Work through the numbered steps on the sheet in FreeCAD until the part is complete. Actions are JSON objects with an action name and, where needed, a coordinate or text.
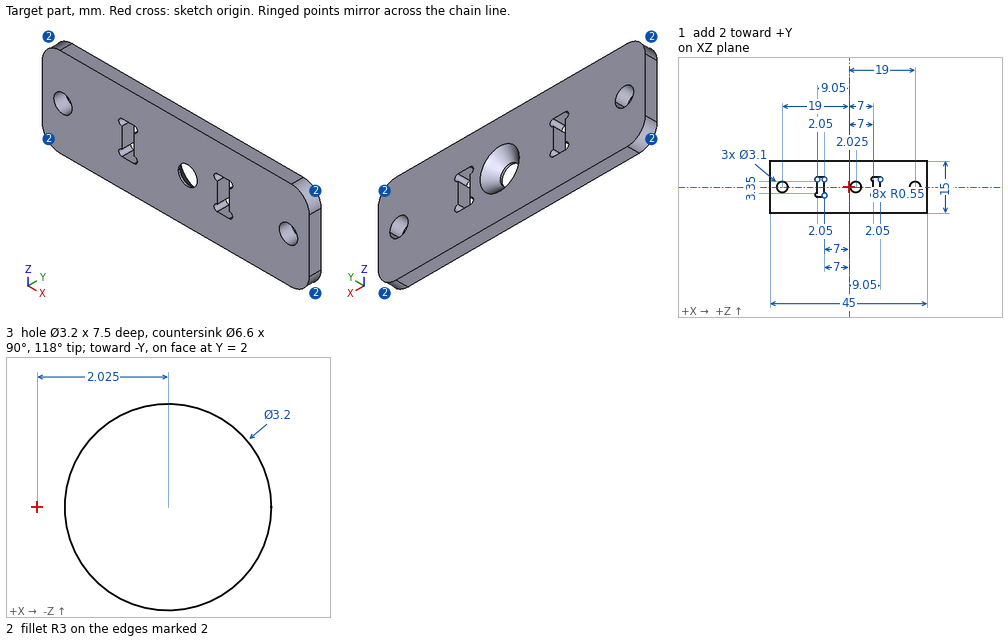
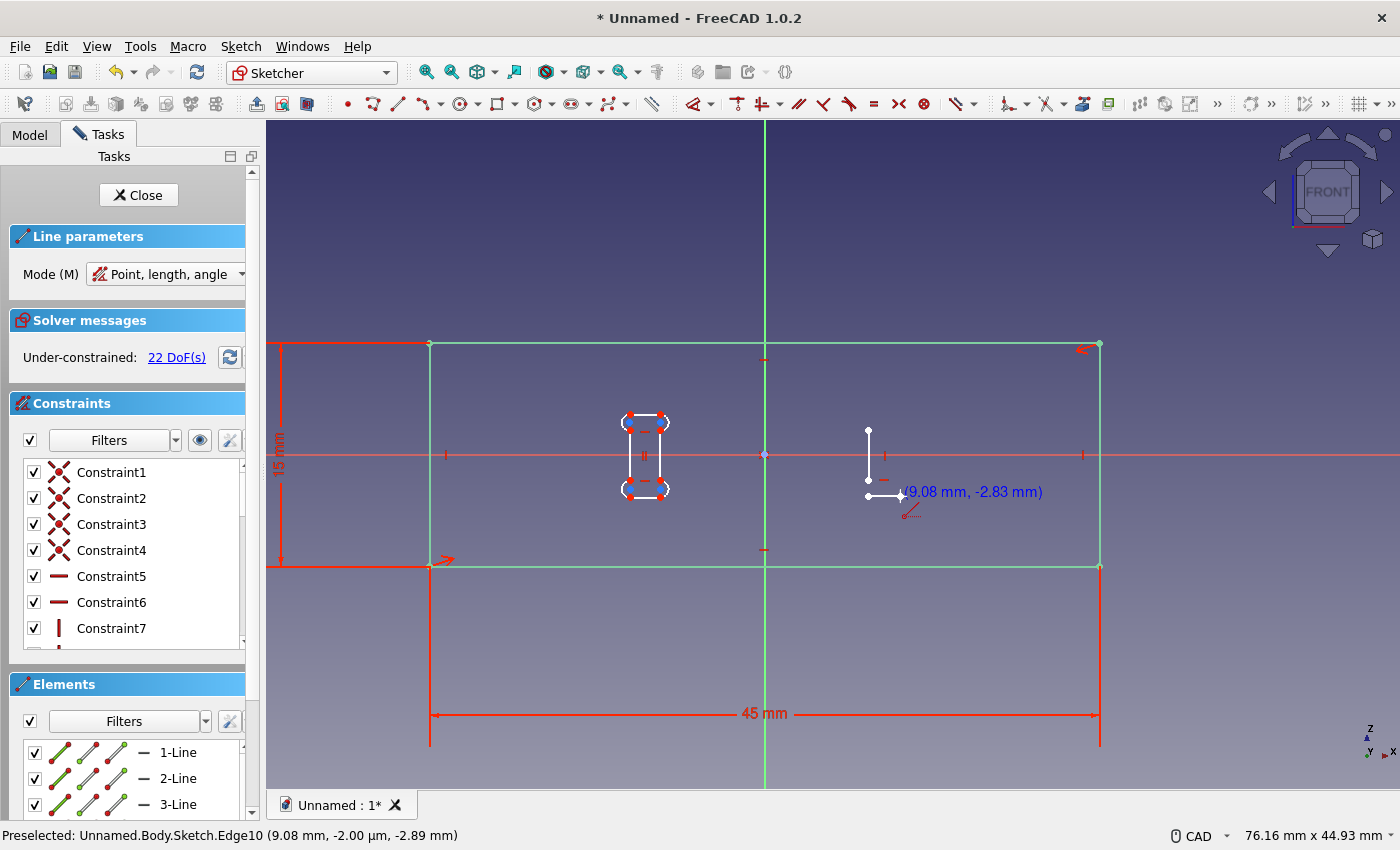
{"action": "left_click", "coordinate": [900, 480]}
{"action": "left_click", "coordinate": [900, 430]}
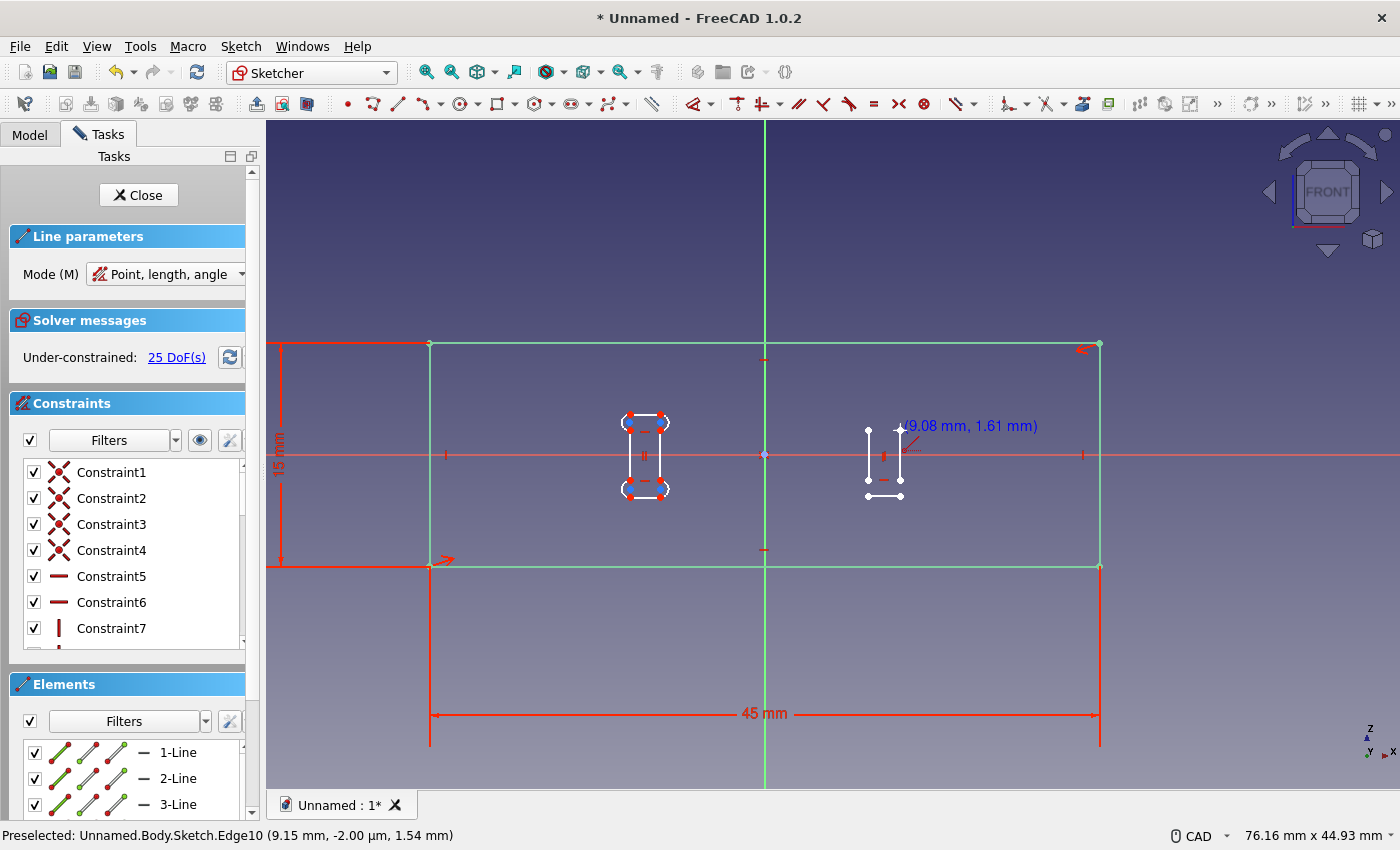
{"action": "left_click", "coordinate": [900, 414]}
{"action": "left_click", "coordinate": [869, 414]}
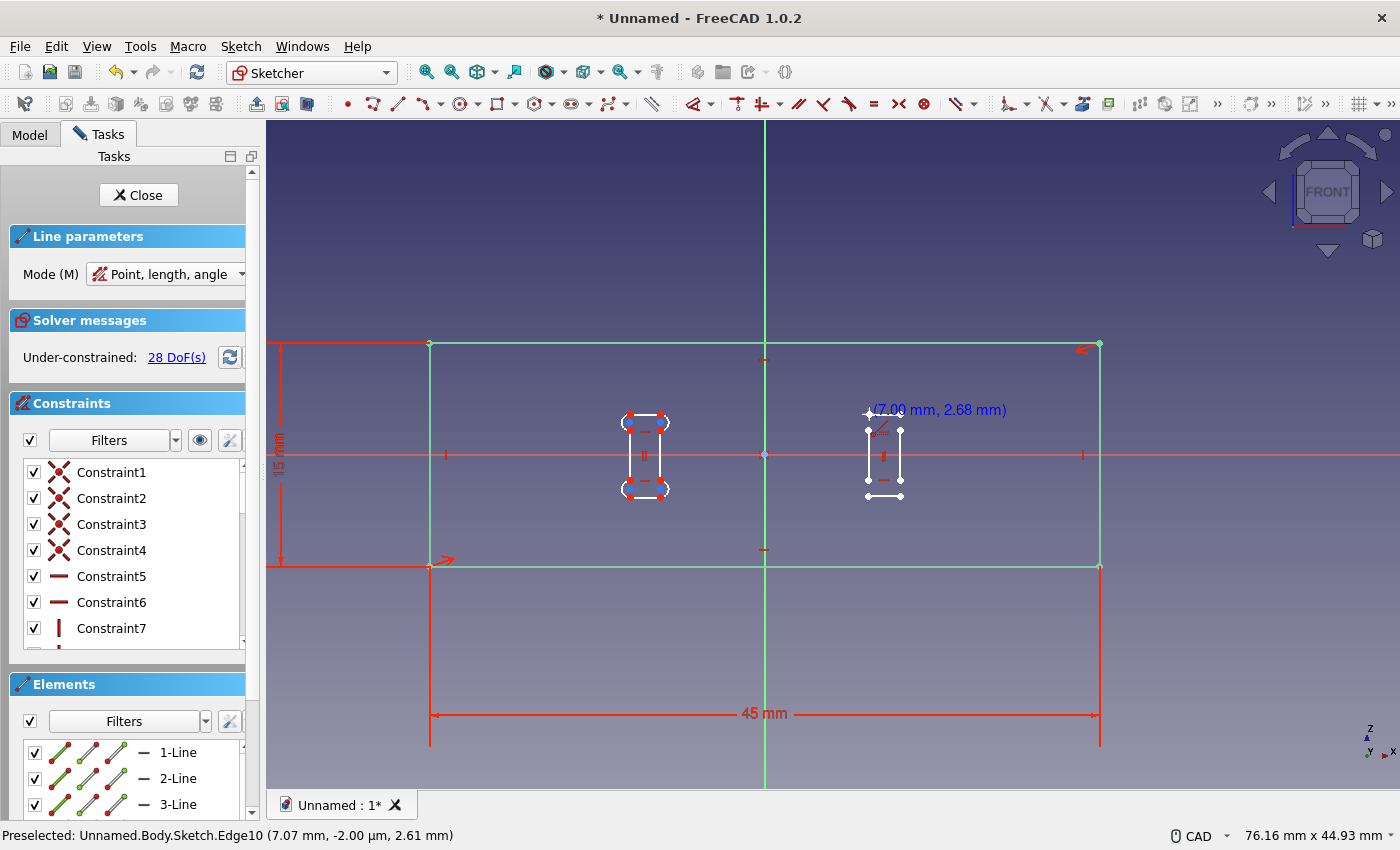
{"action": "left_click", "coordinate": [422, 104]}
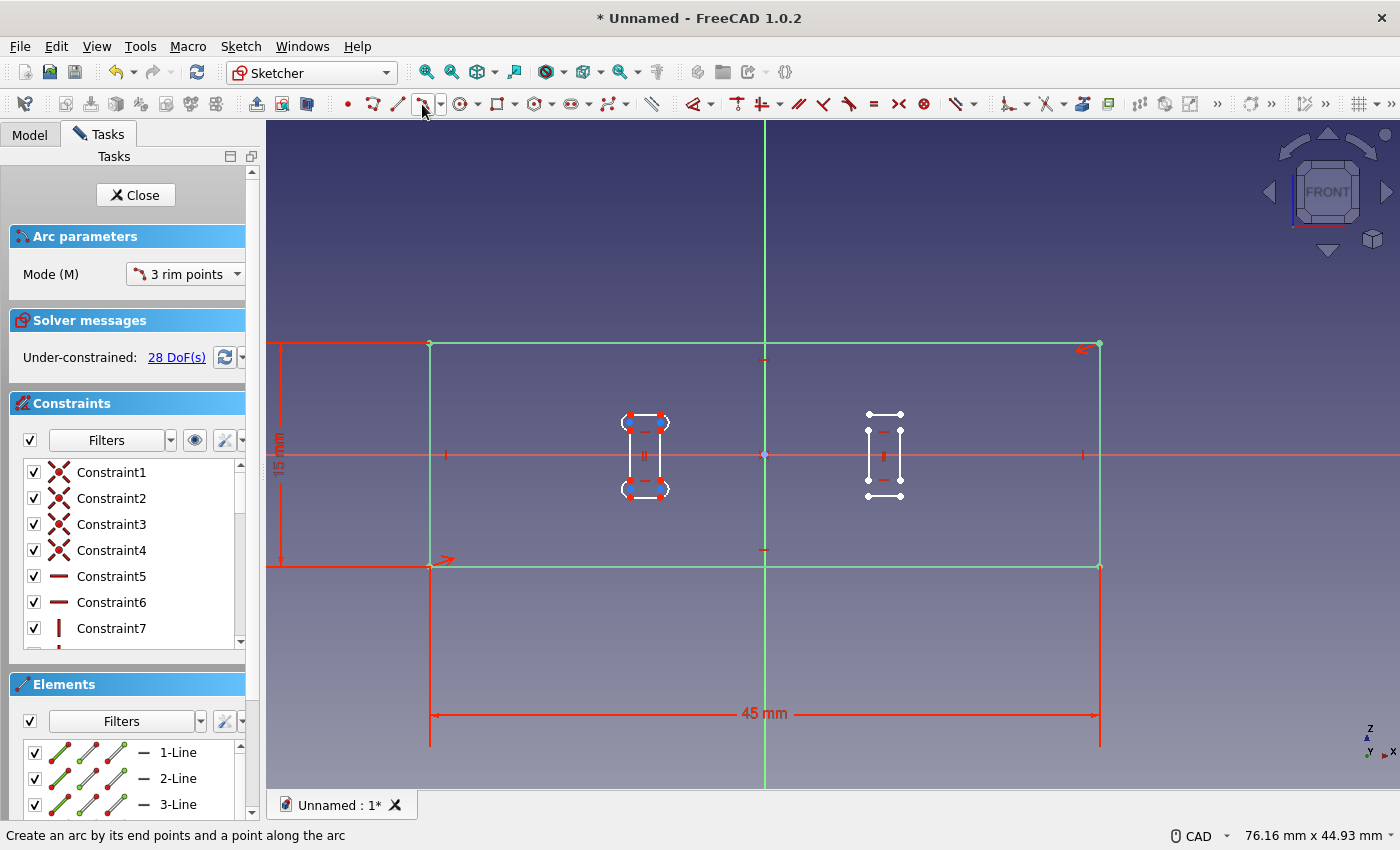
{"action": "left_click", "coordinate": [869, 480]}
{"action": "left_click", "coordinate": [869, 496]}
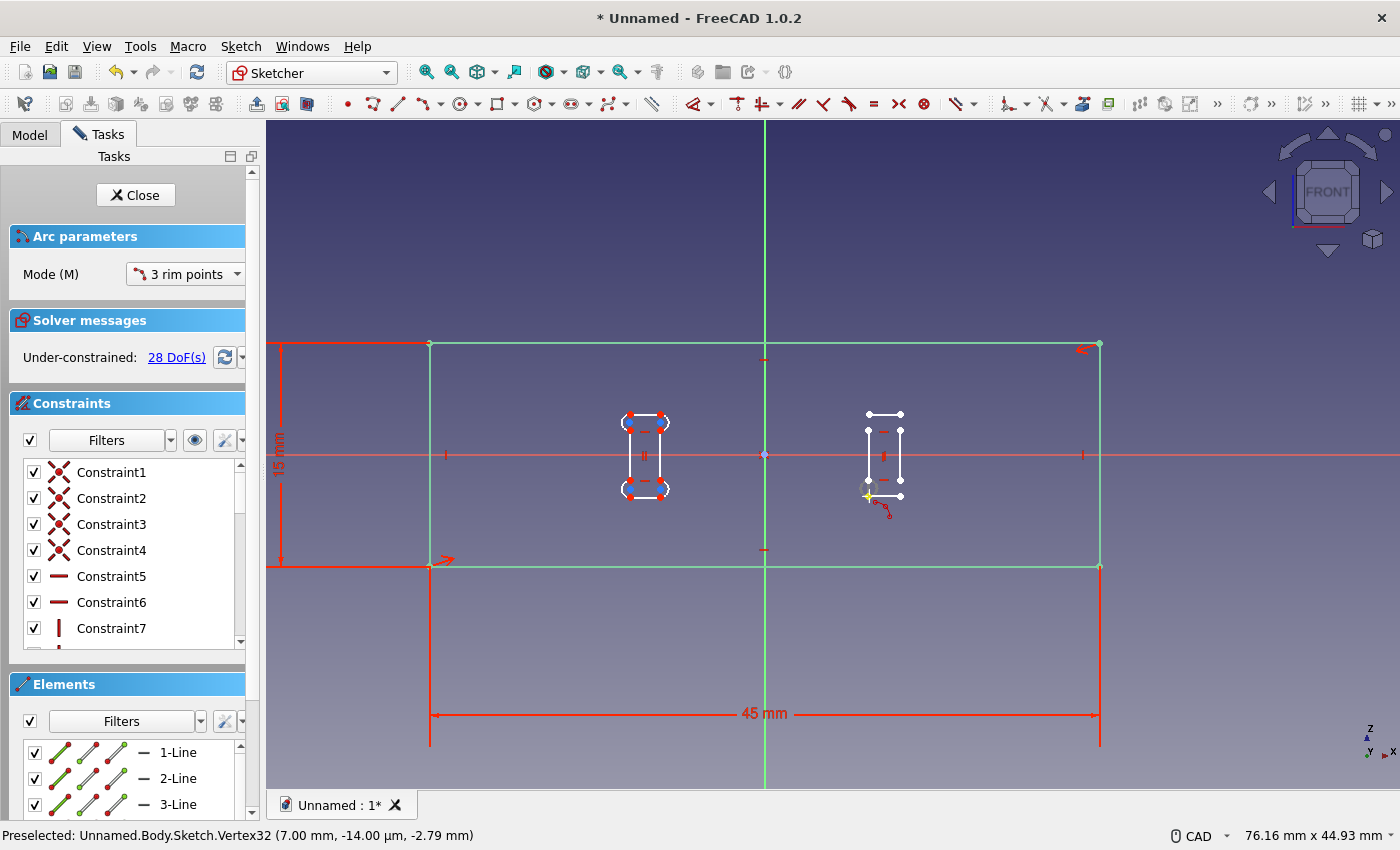
{"action": "scroll", "coordinate": [861, 488], "scroll_direction": "up", "scroll_amount": 4}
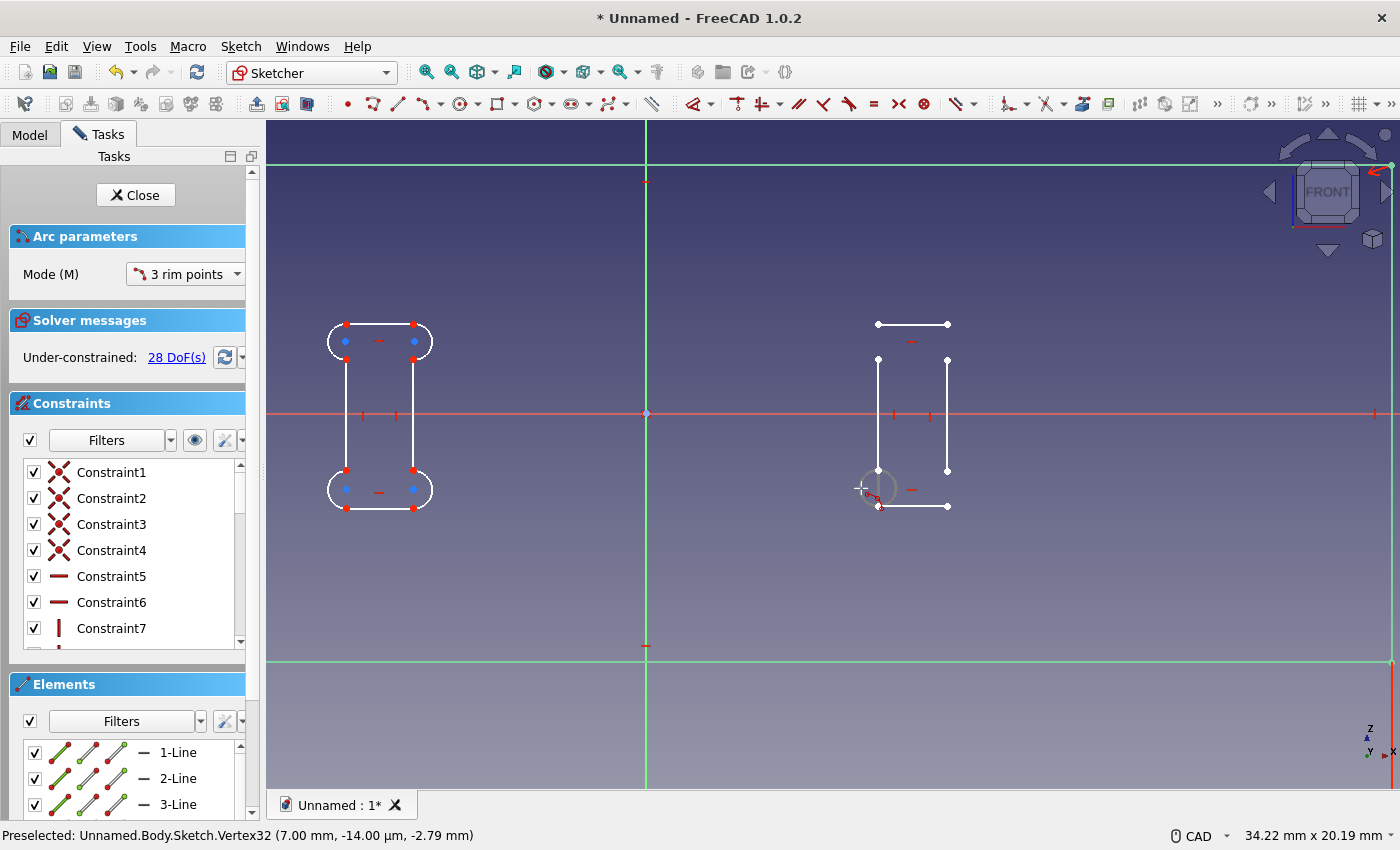
{"action": "left_click", "coordinate": [860, 487]}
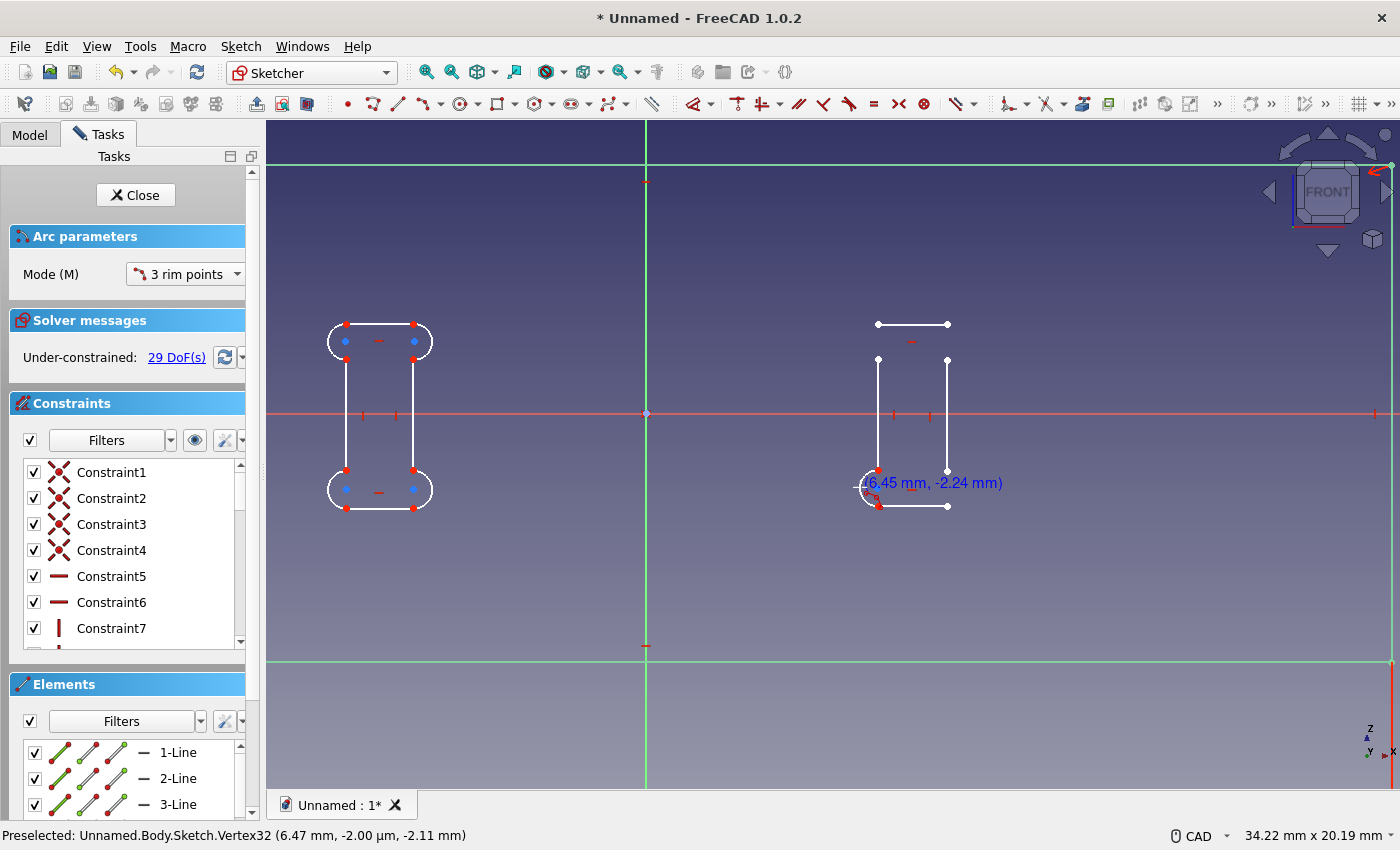
{"action": "left_click", "coordinate": [947, 506]}
{"action": "left_click", "coordinate": [947, 472]}
{"action": "left_click", "coordinate": [964, 487]}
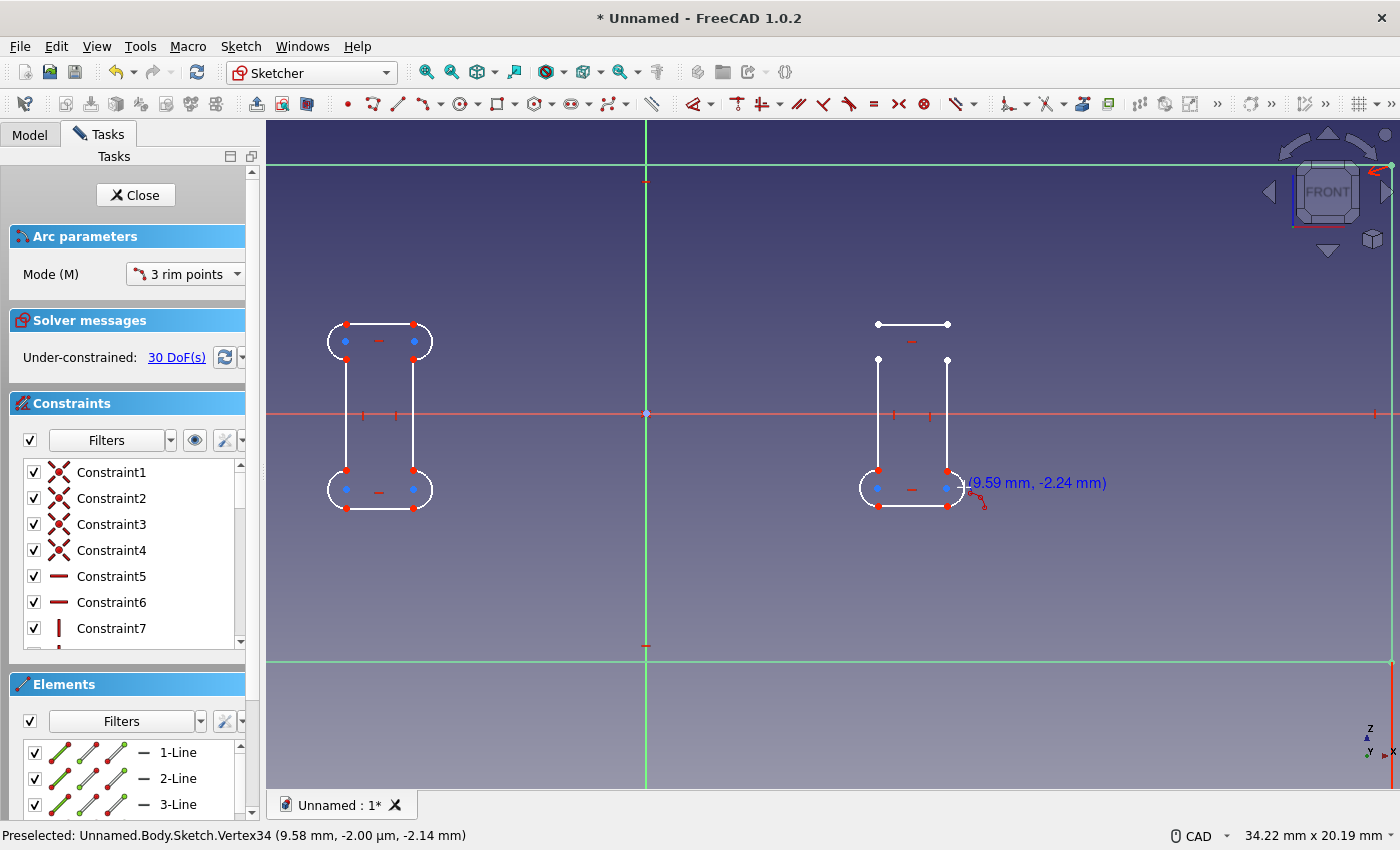
{"action": "left_click", "coordinate": [947, 360]}
{"action": "left_click", "coordinate": [947, 325]}
{"action": "left_click", "coordinate": [964, 340]}